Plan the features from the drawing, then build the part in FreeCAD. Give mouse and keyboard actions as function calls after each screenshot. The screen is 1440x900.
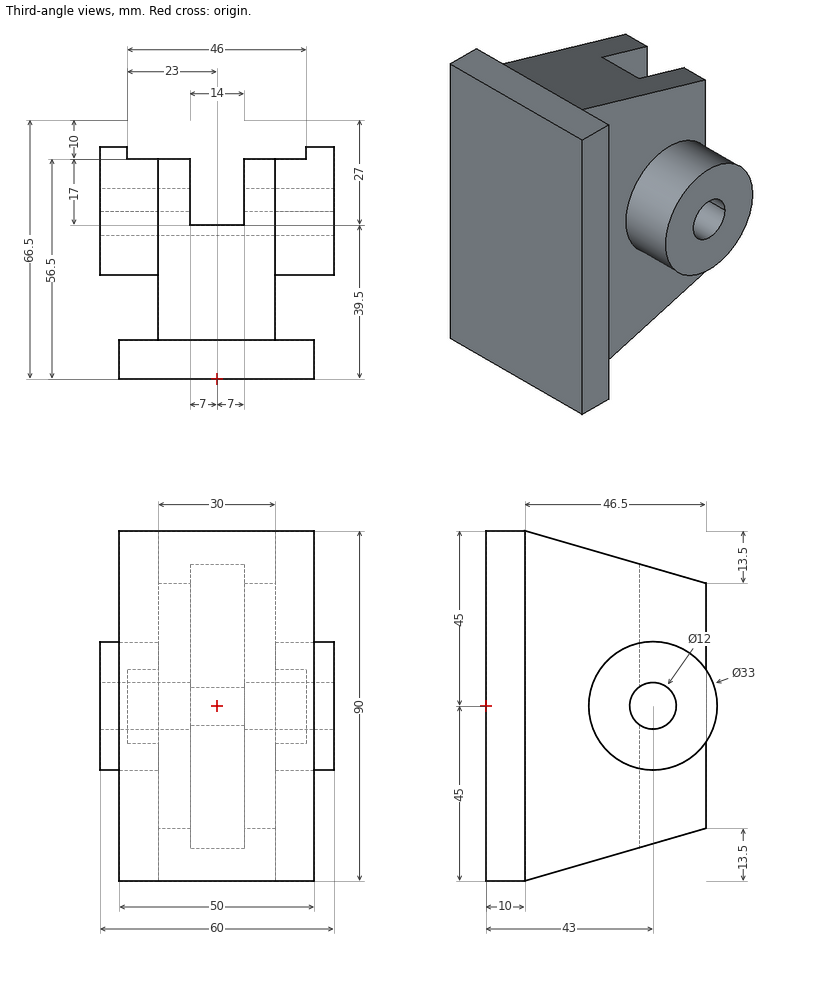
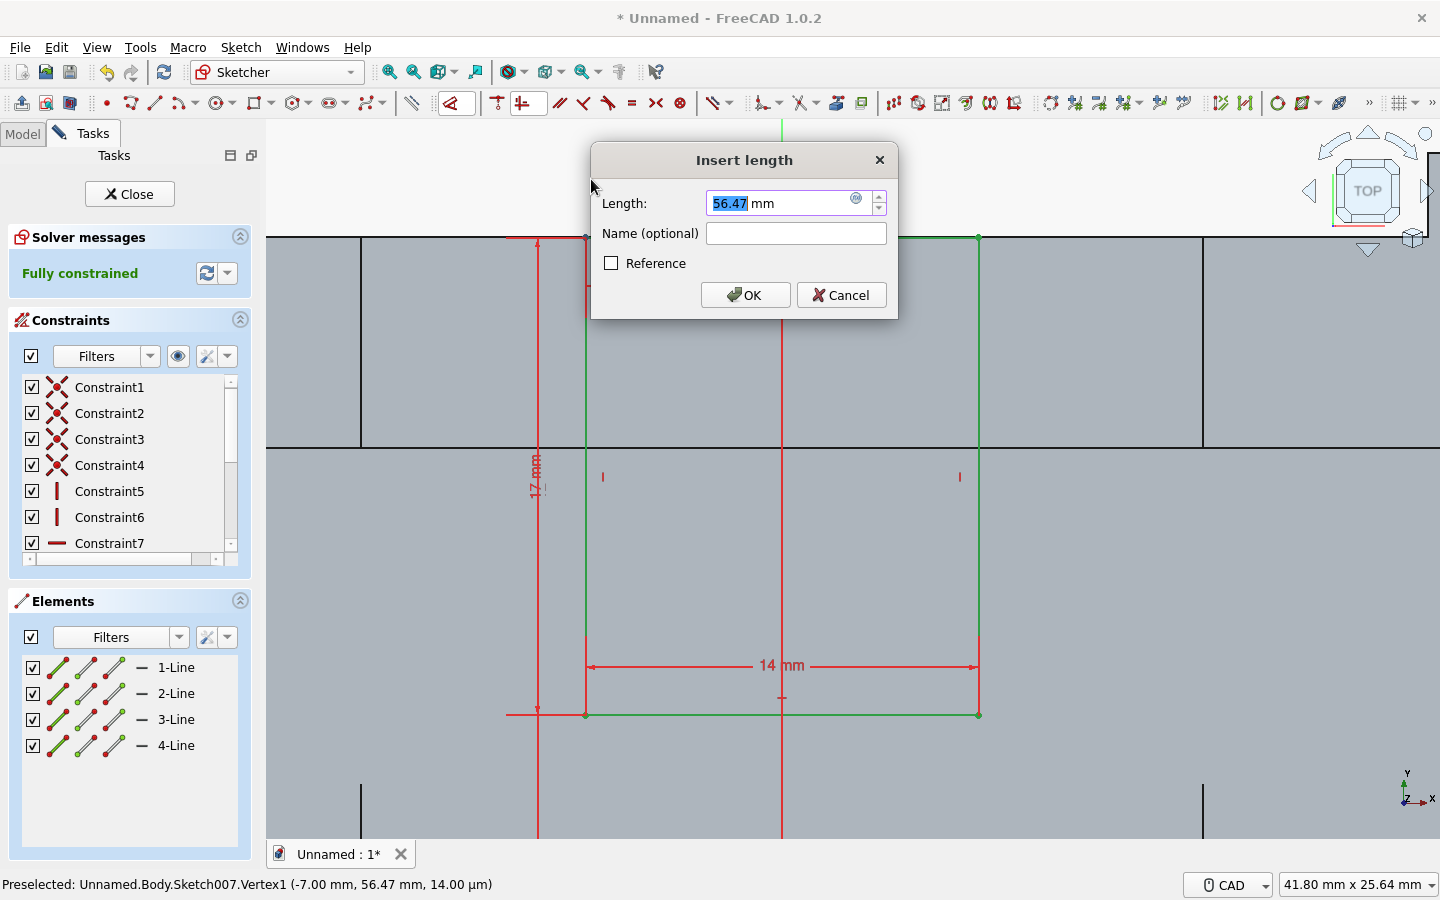
text(56.5)
key(Return)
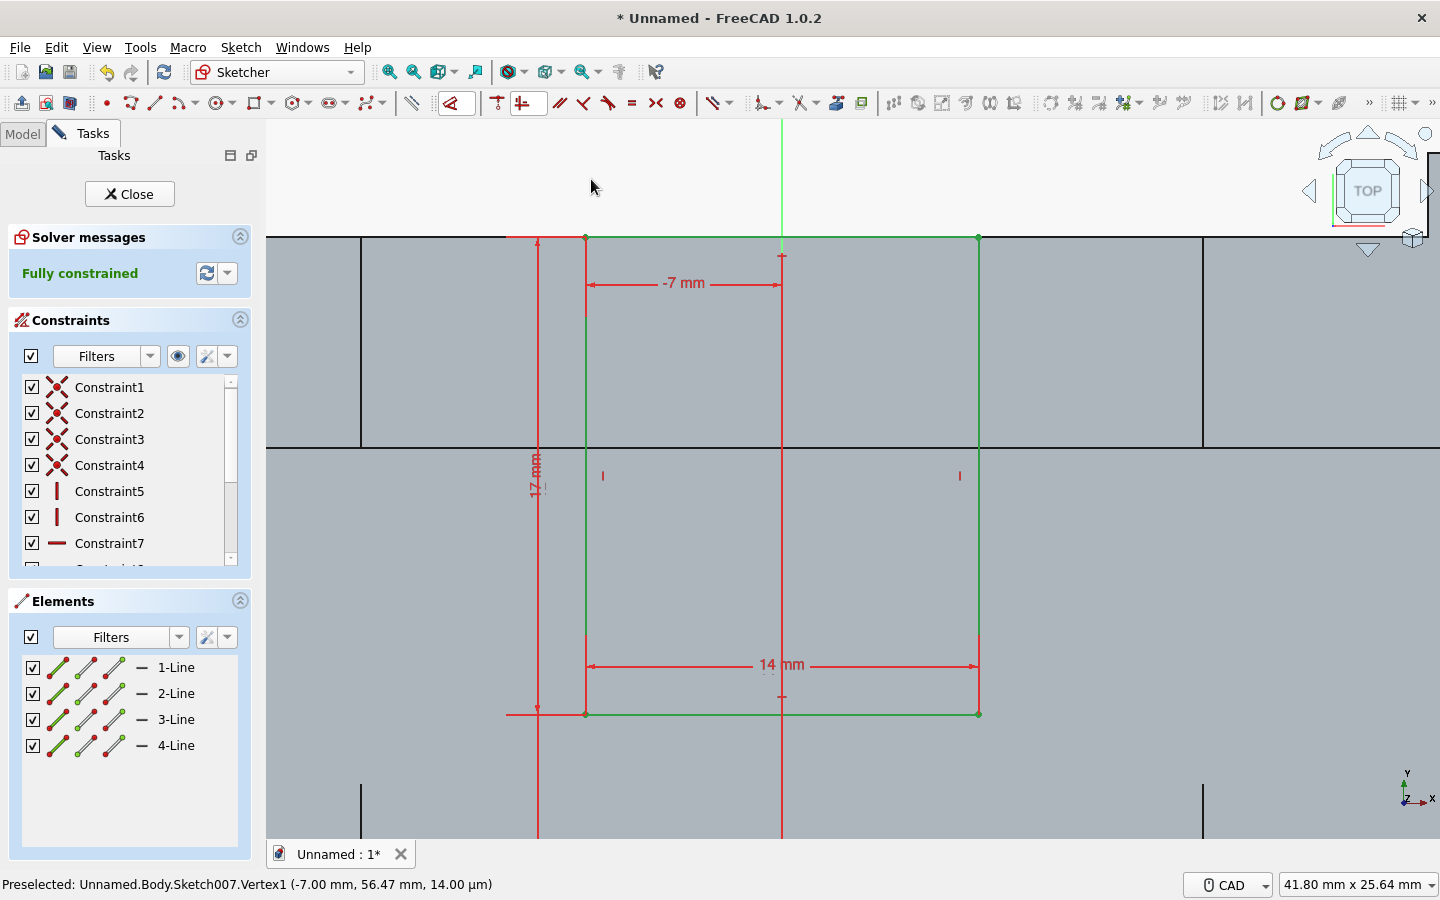
click(130, 194)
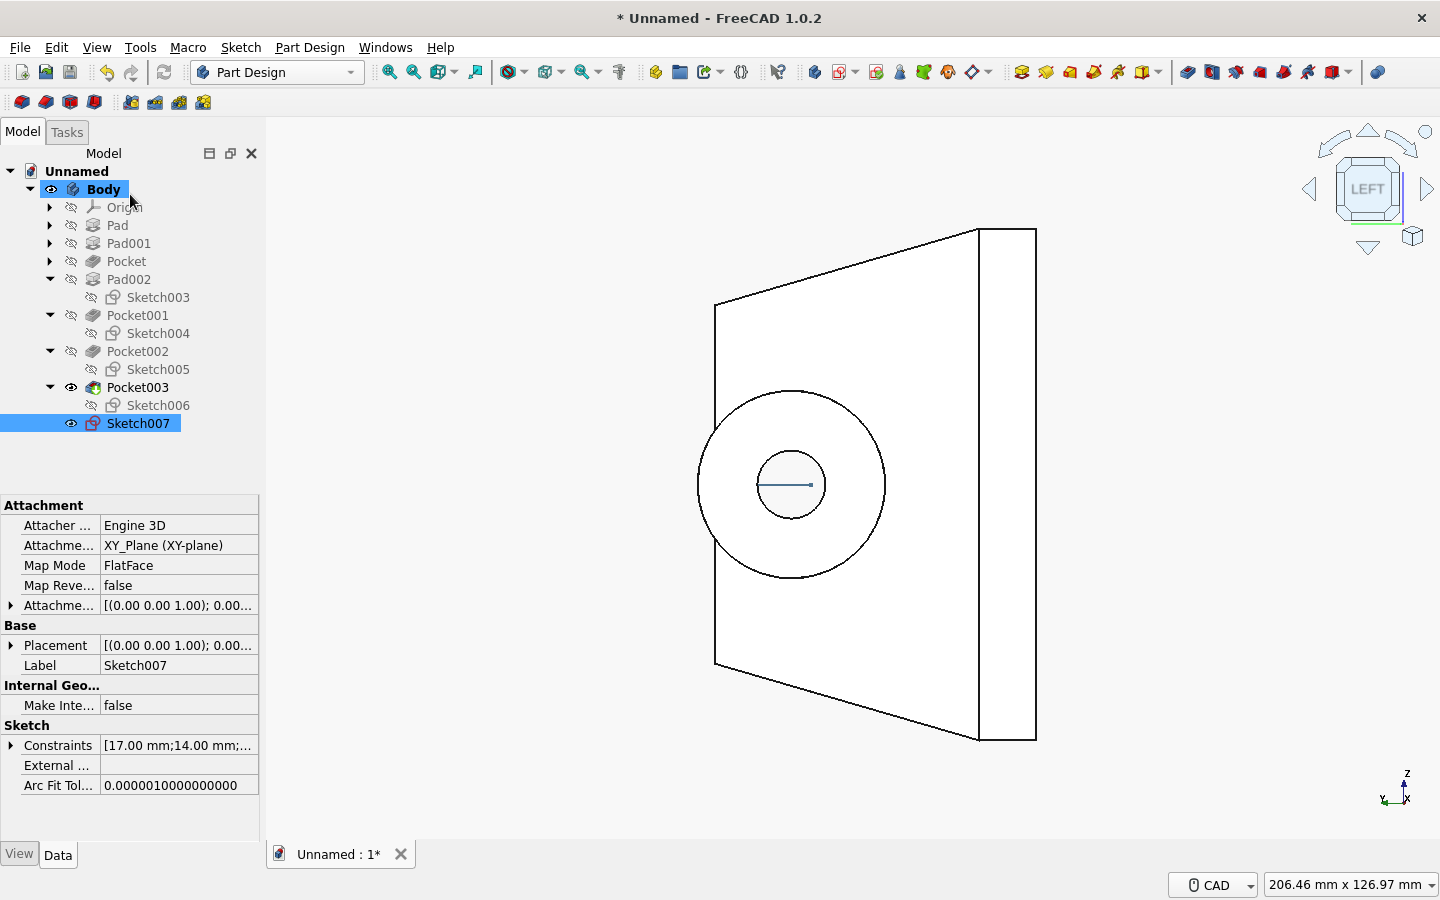
click(1188, 72)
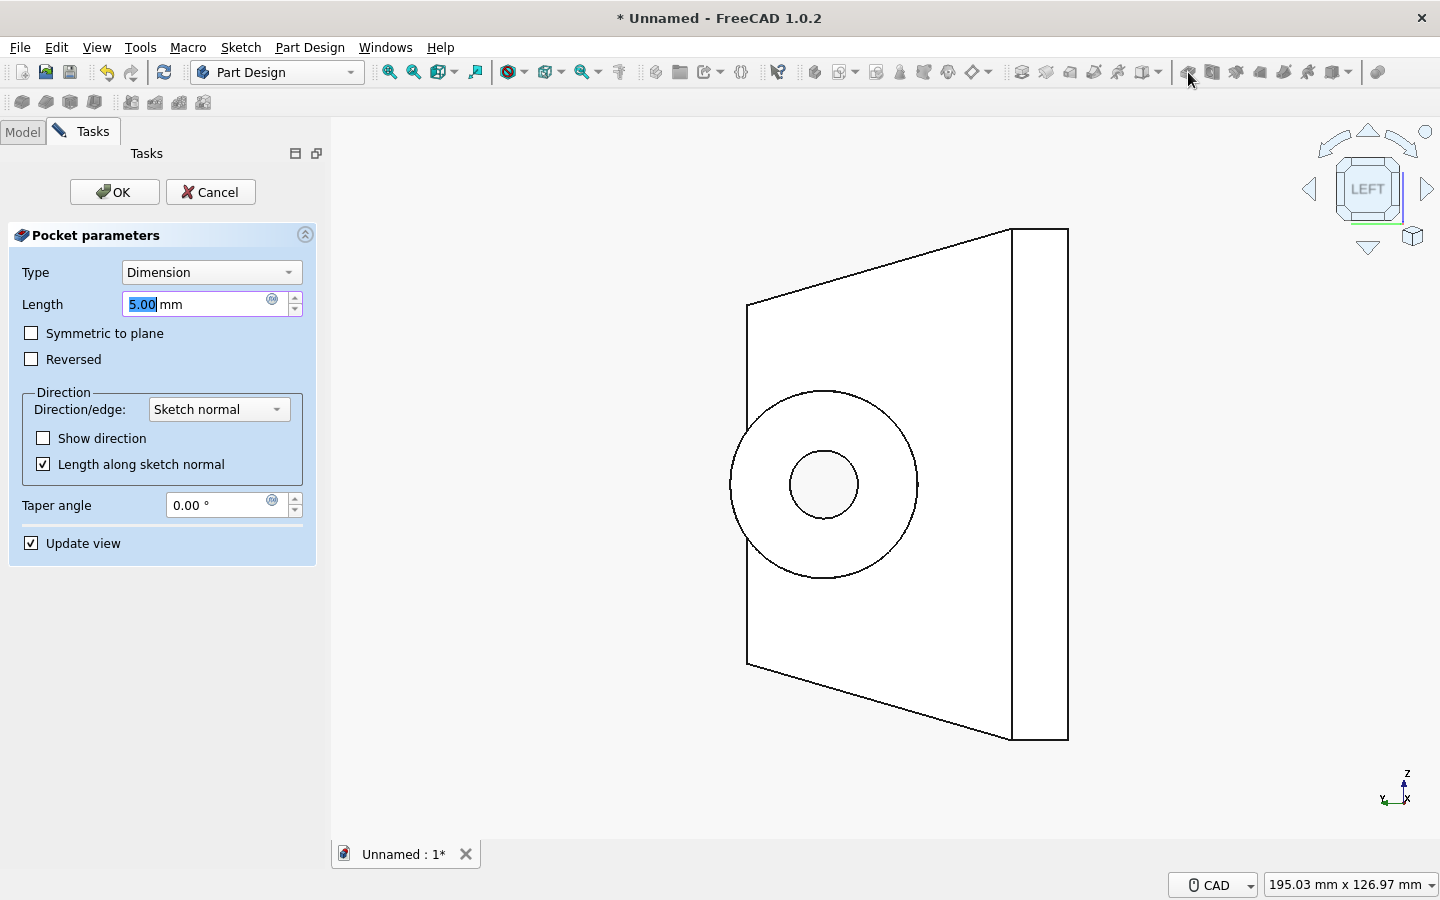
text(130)
key(Tab)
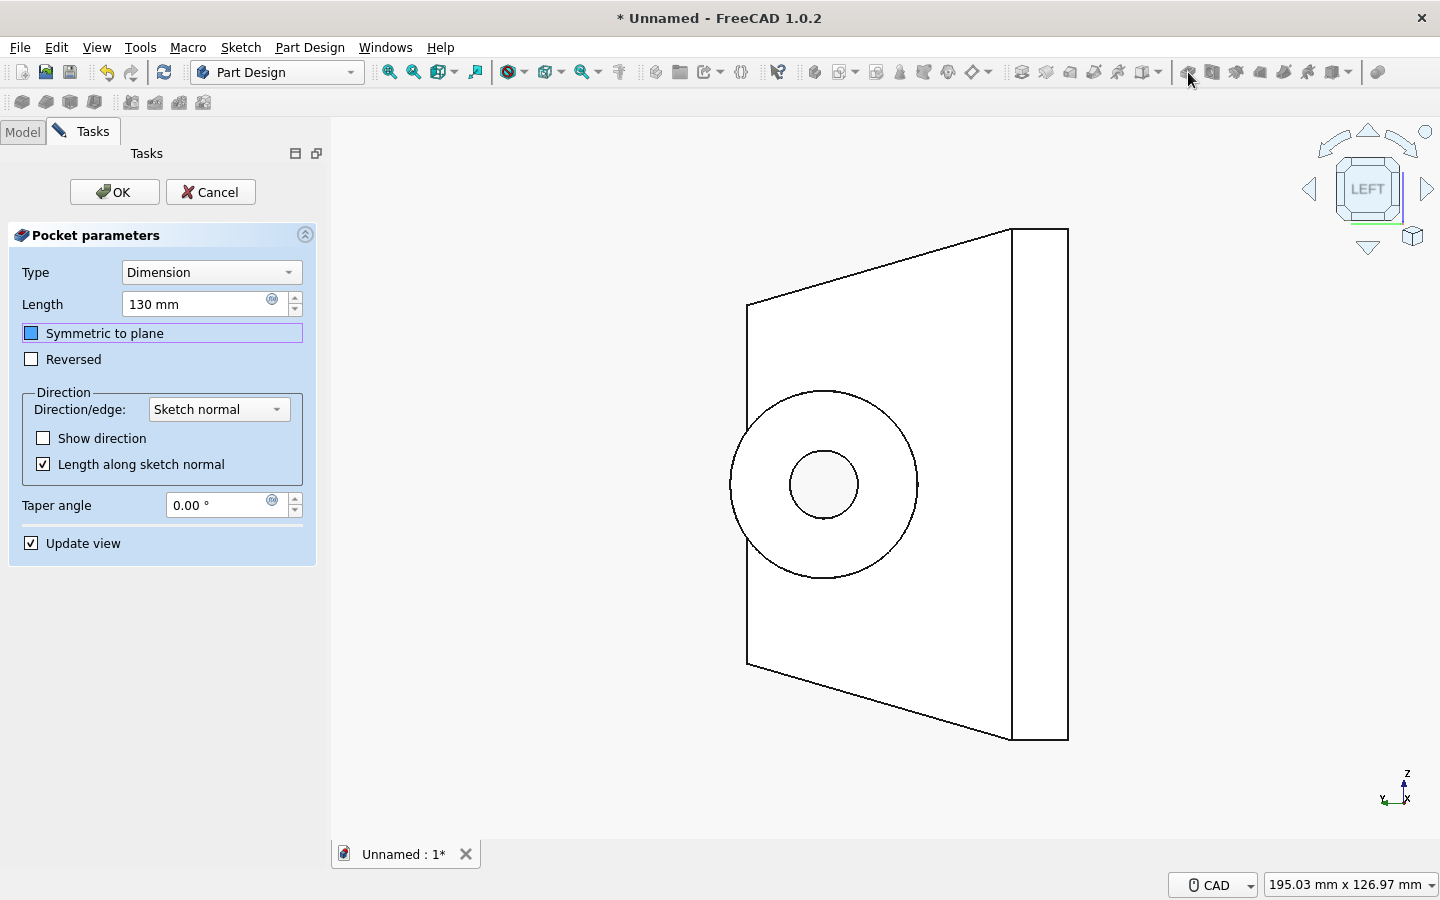
click(30, 333)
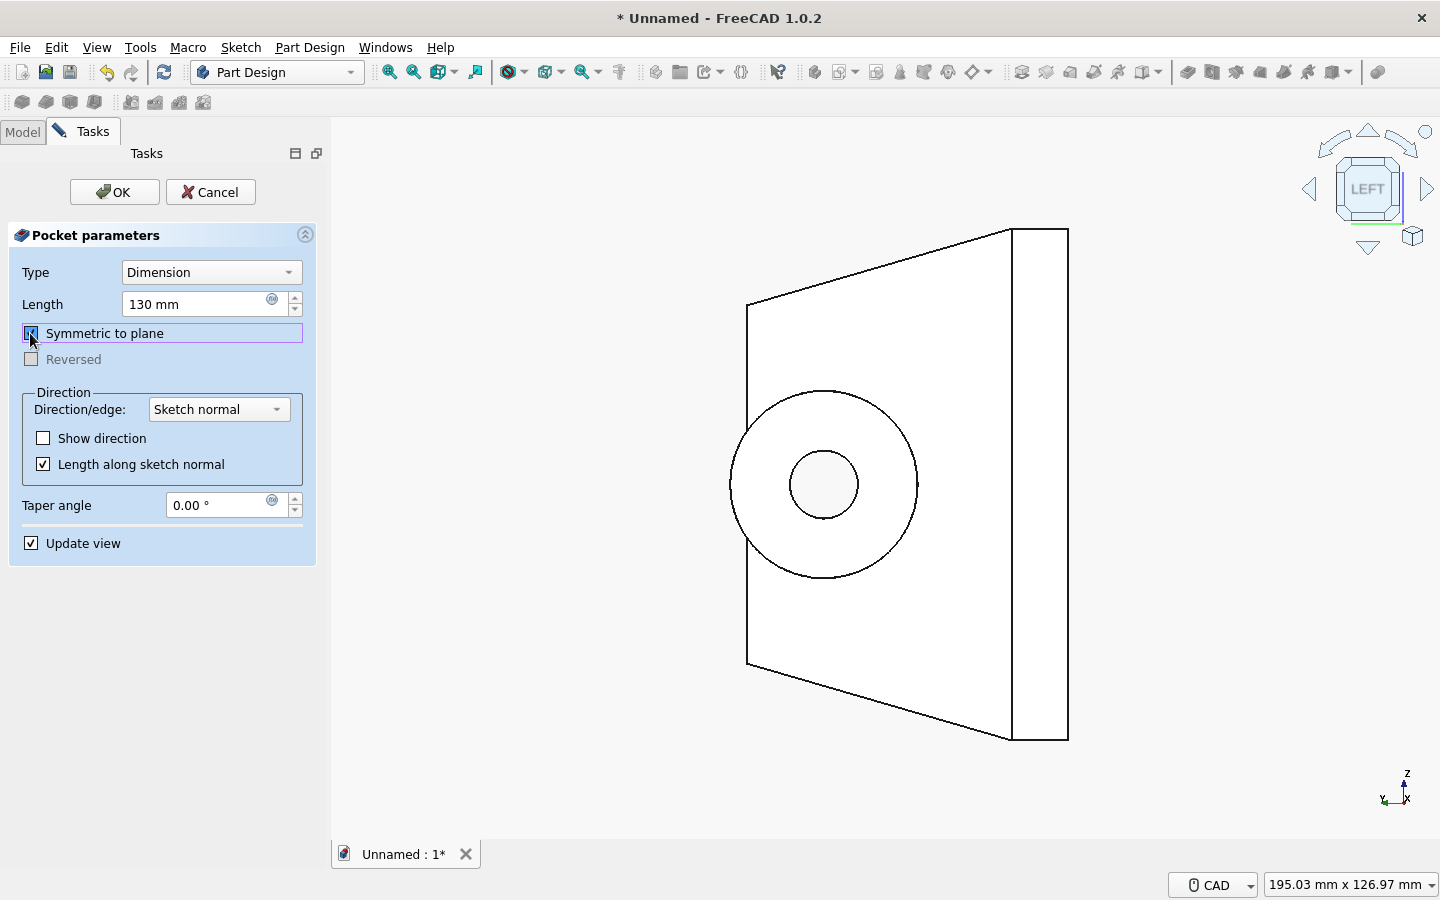
click(115, 192)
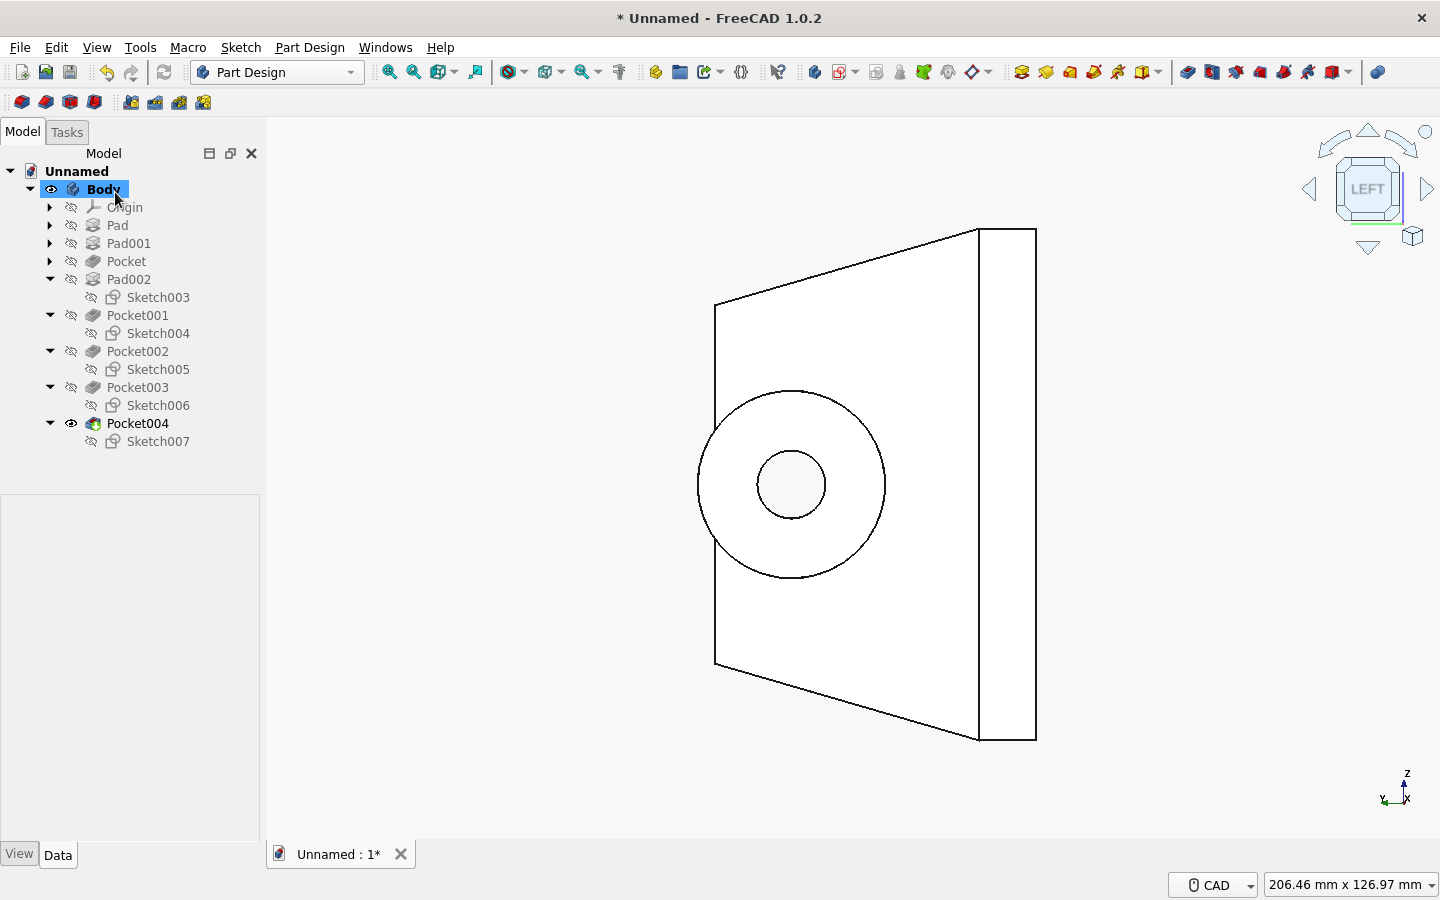
key(0)